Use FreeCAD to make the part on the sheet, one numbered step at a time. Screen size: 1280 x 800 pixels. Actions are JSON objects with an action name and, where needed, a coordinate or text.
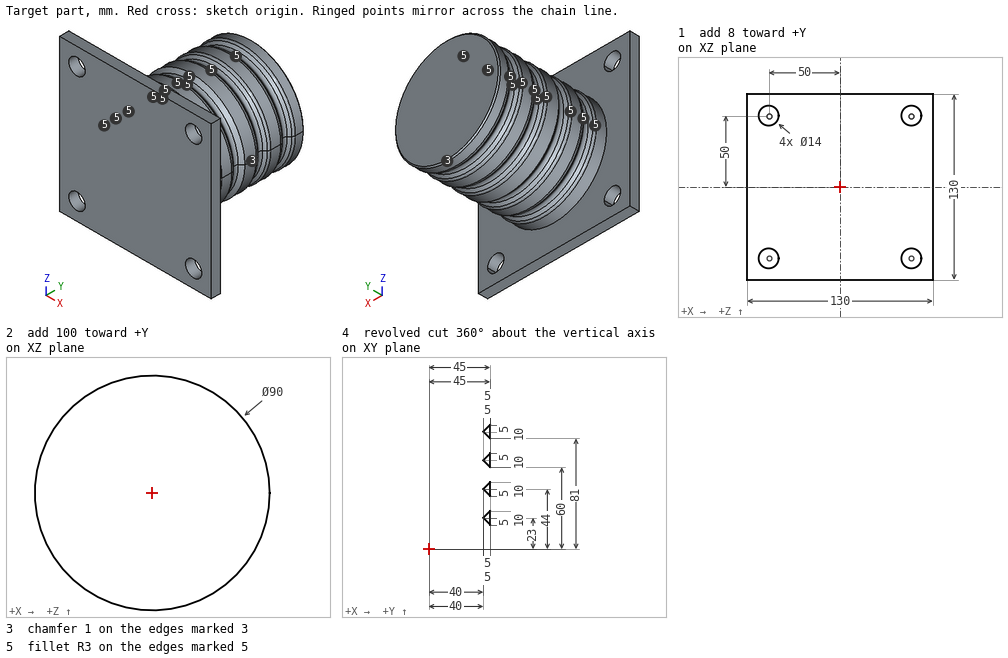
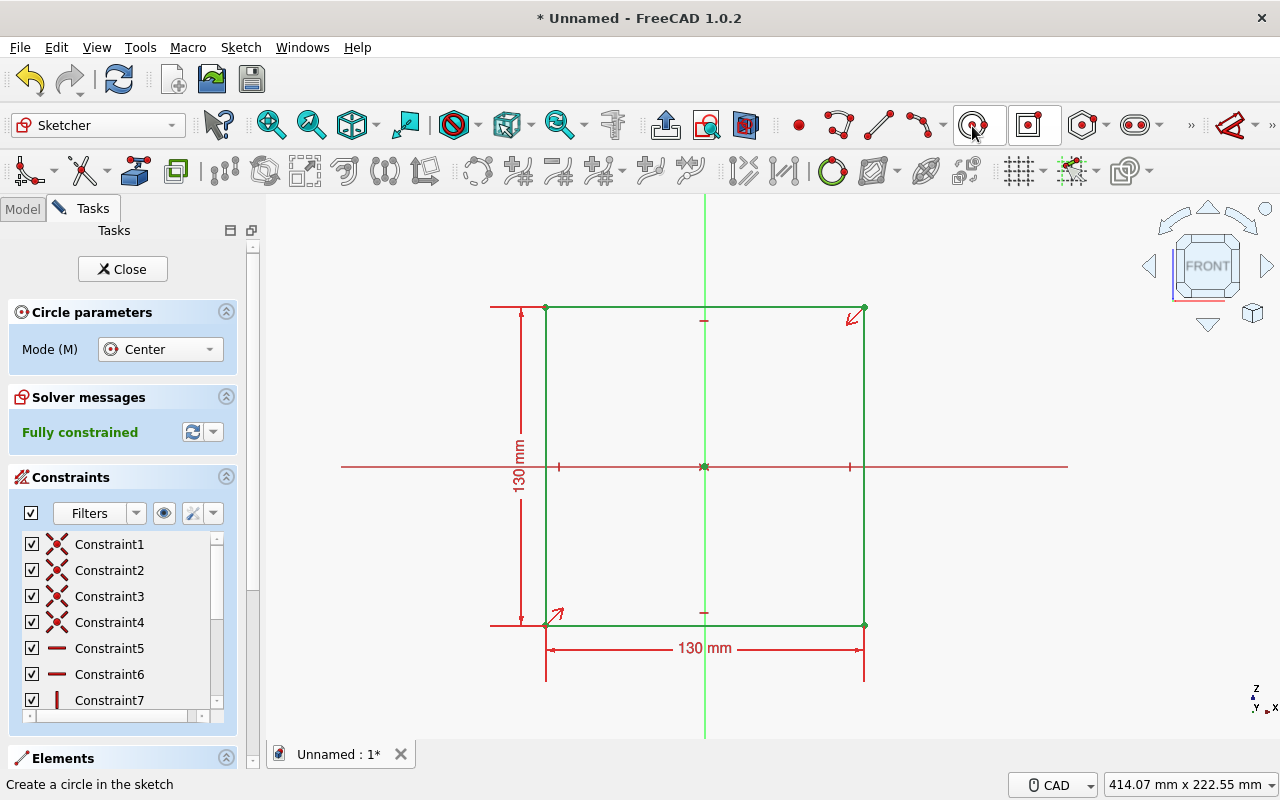
{"action": "scroll", "coordinate": [582, 344], "scroll_direction": "up", "scroll_amount": 2}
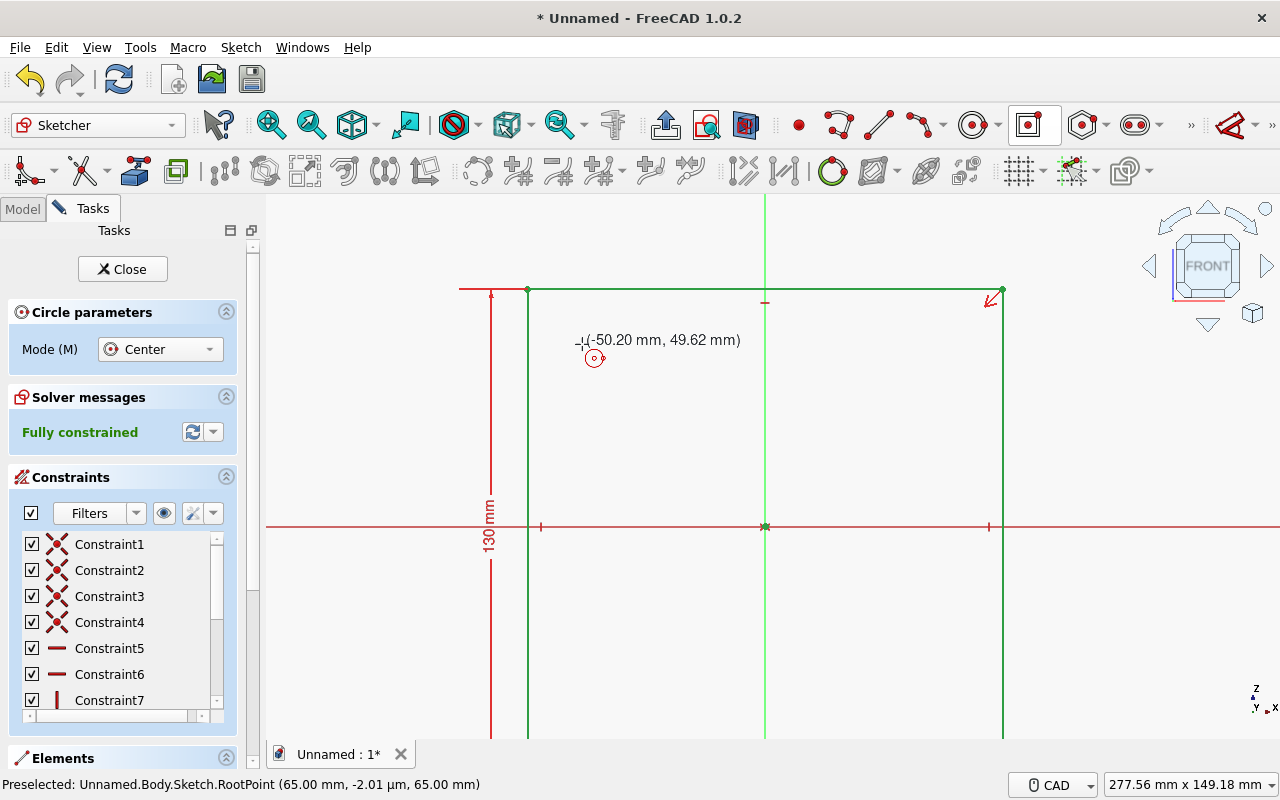
{"action": "left_click", "coordinate": [583, 344]}
{"action": "mouse_move", "coordinate": [601, 326]}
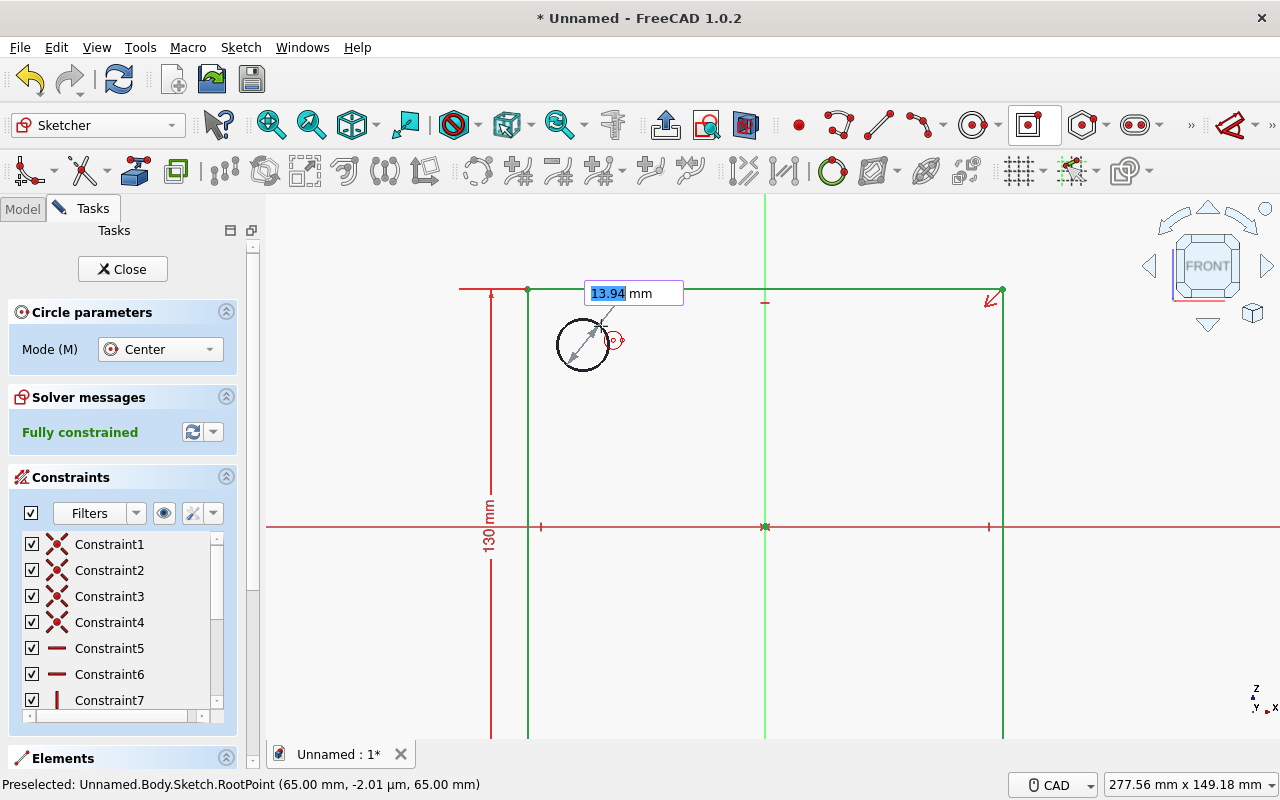
{"action": "type", "text": "14"}
{"action": "key", "text": "Return"}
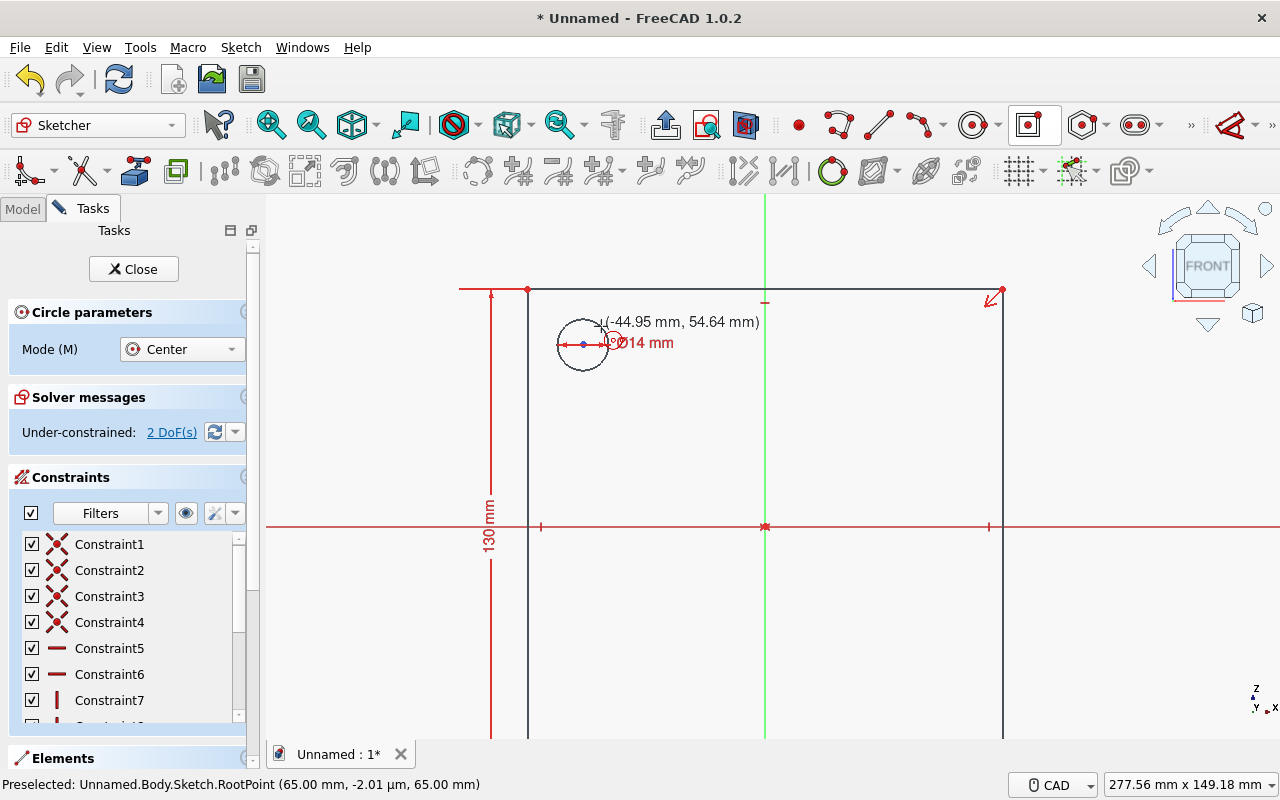
{"action": "left_click", "coordinate": [948, 344]}
{"action": "mouse_move", "coordinate": [966, 326]}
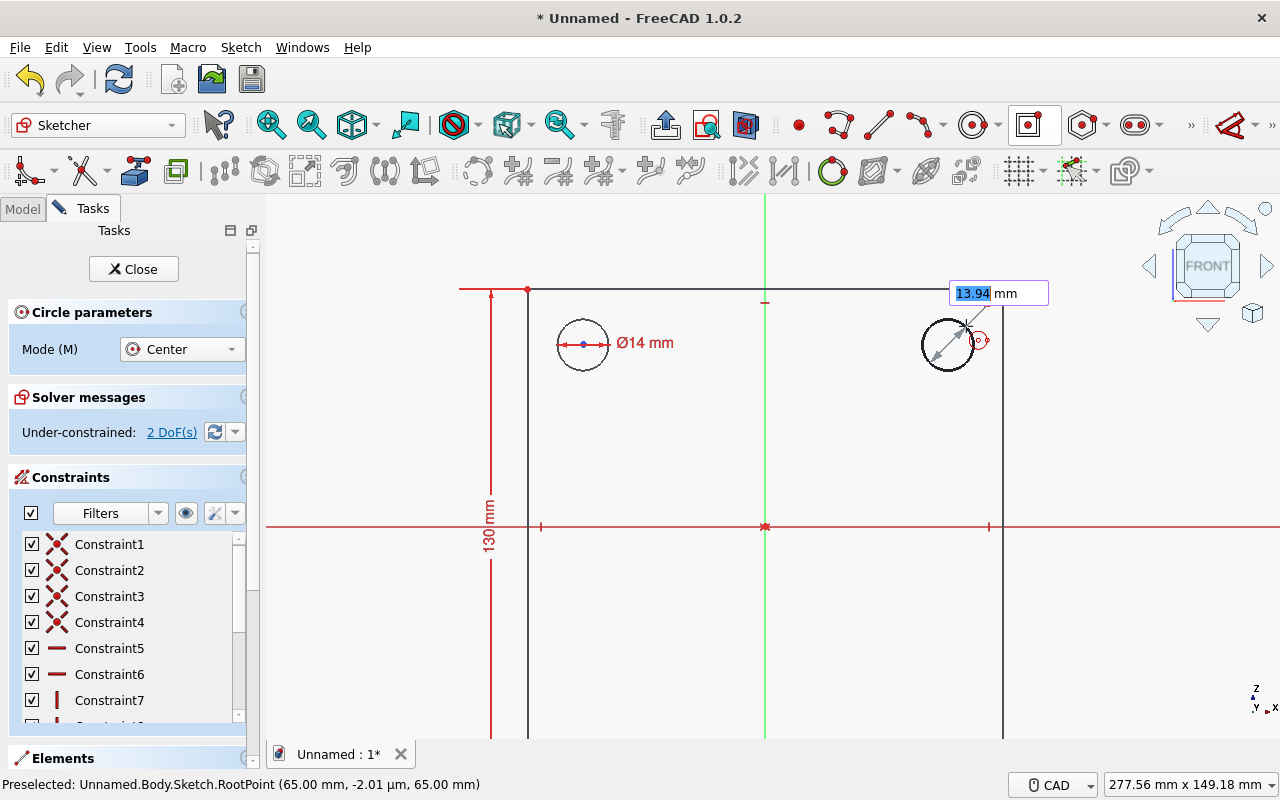
{"action": "type", "text": "14"}
{"action": "key", "text": "Return"}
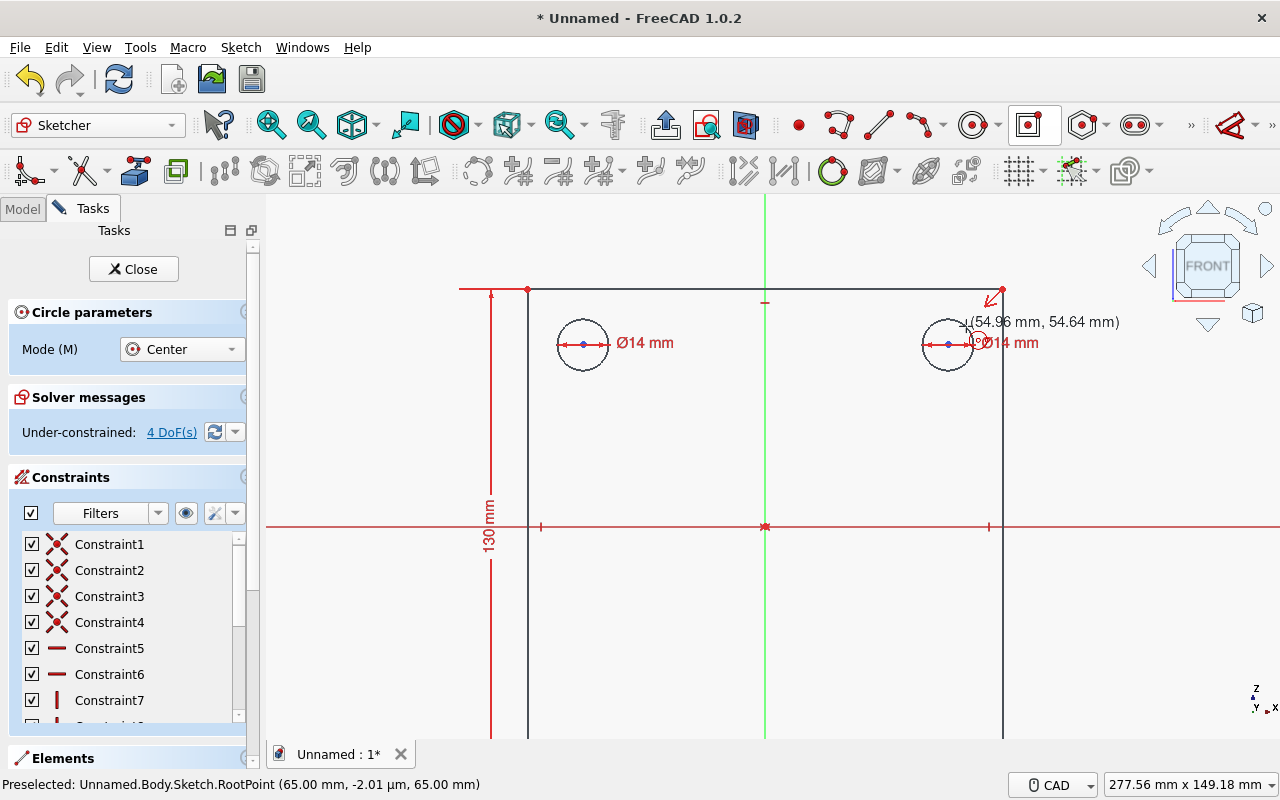
{"action": "left_click", "coordinate": [583, 709]}
{"action": "mouse_move", "coordinate": [601, 691]}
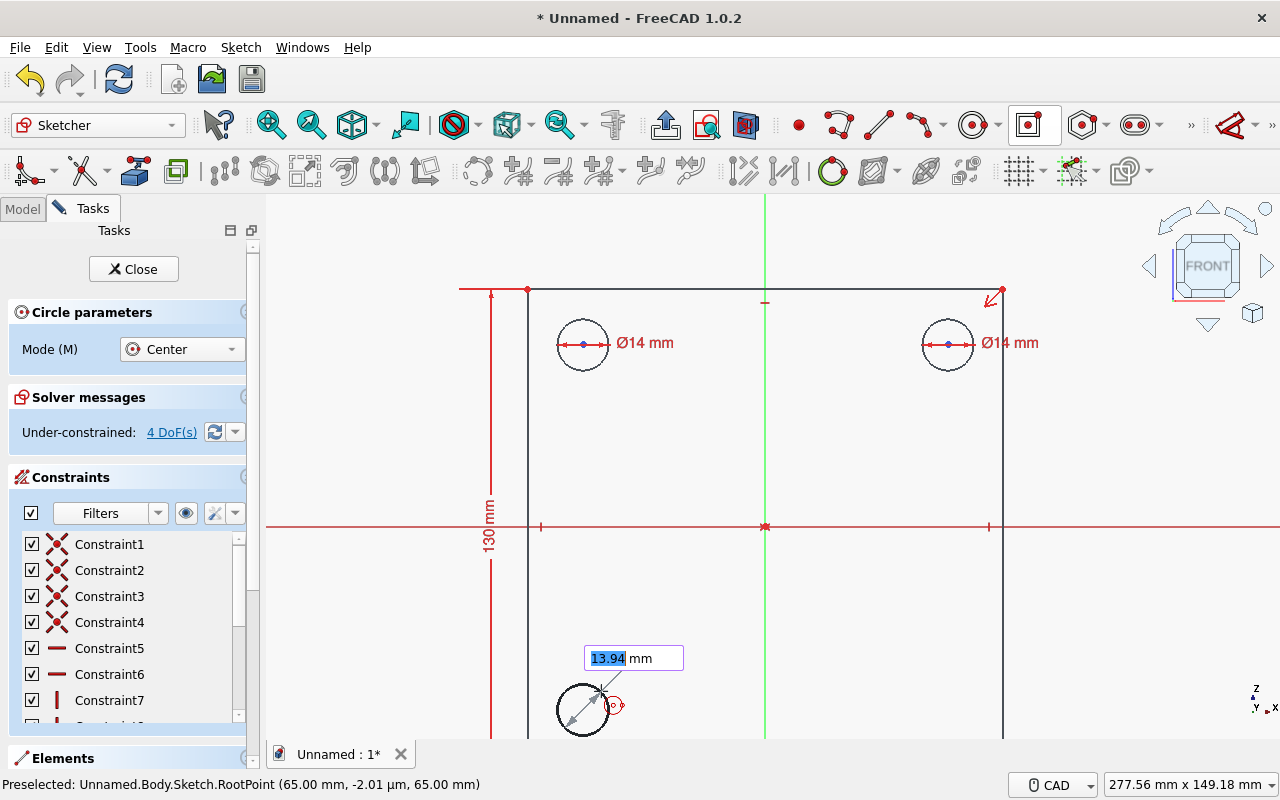
{"action": "type", "text": "14"}
{"action": "key", "text": "Return"}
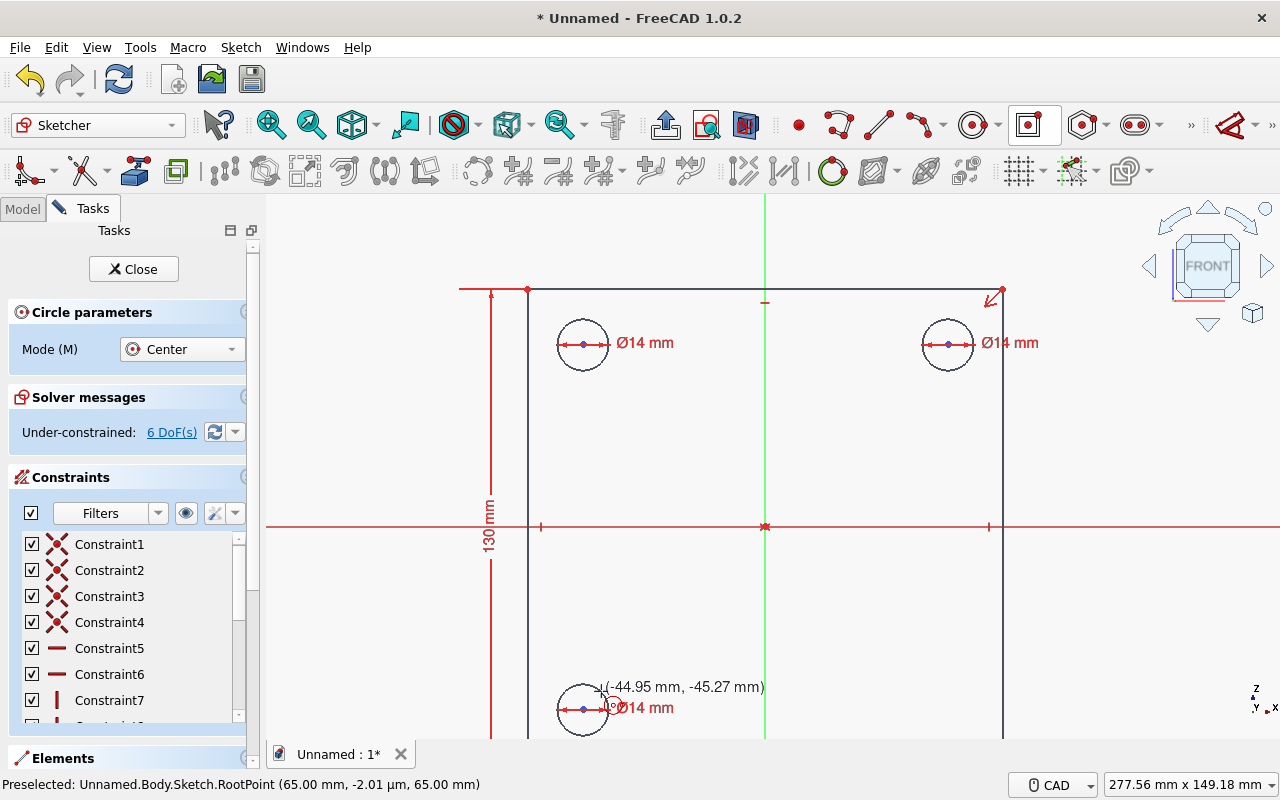
{"action": "left_click", "coordinate": [948, 709]}
{"action": "mouse_move", "coordinate": [966, 691]}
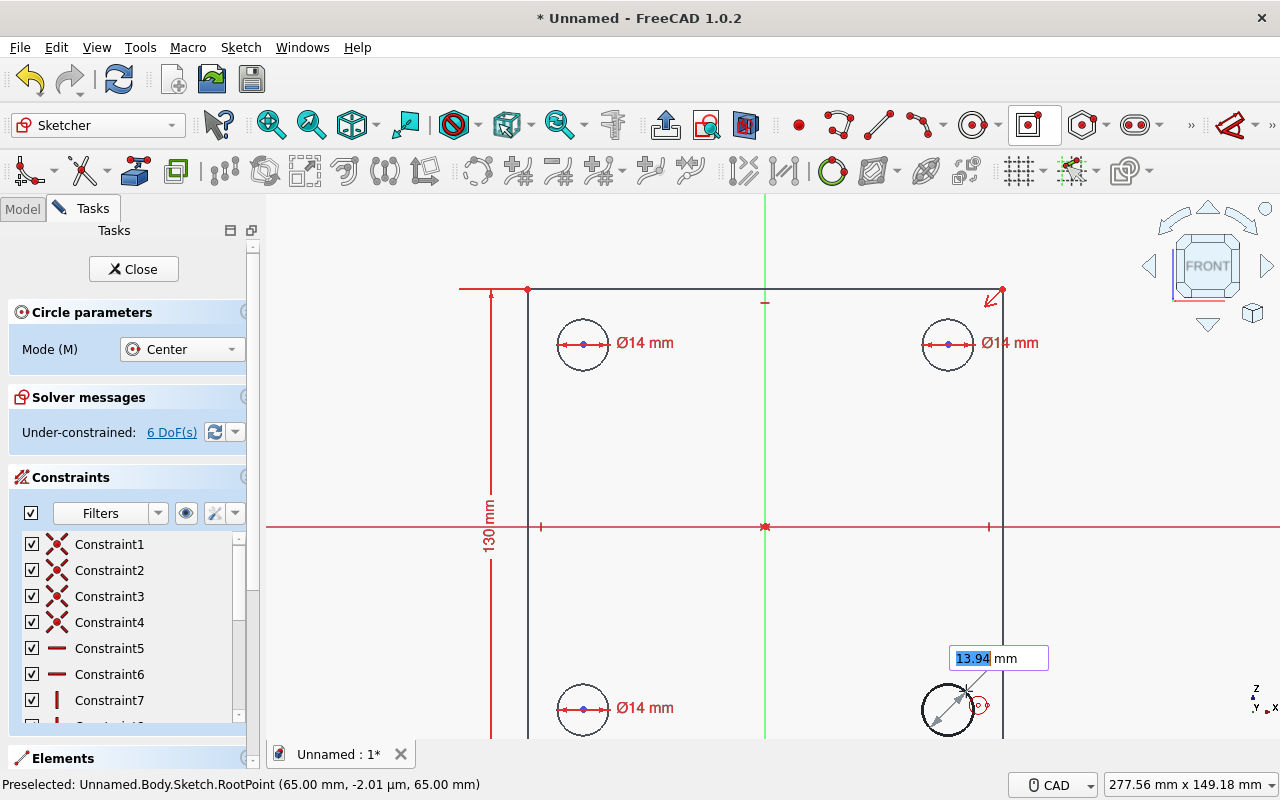
{"action": "type", "text": "14"}
{"action": "key", "text": "Return"}
{"action": "key", "text": "Escape"}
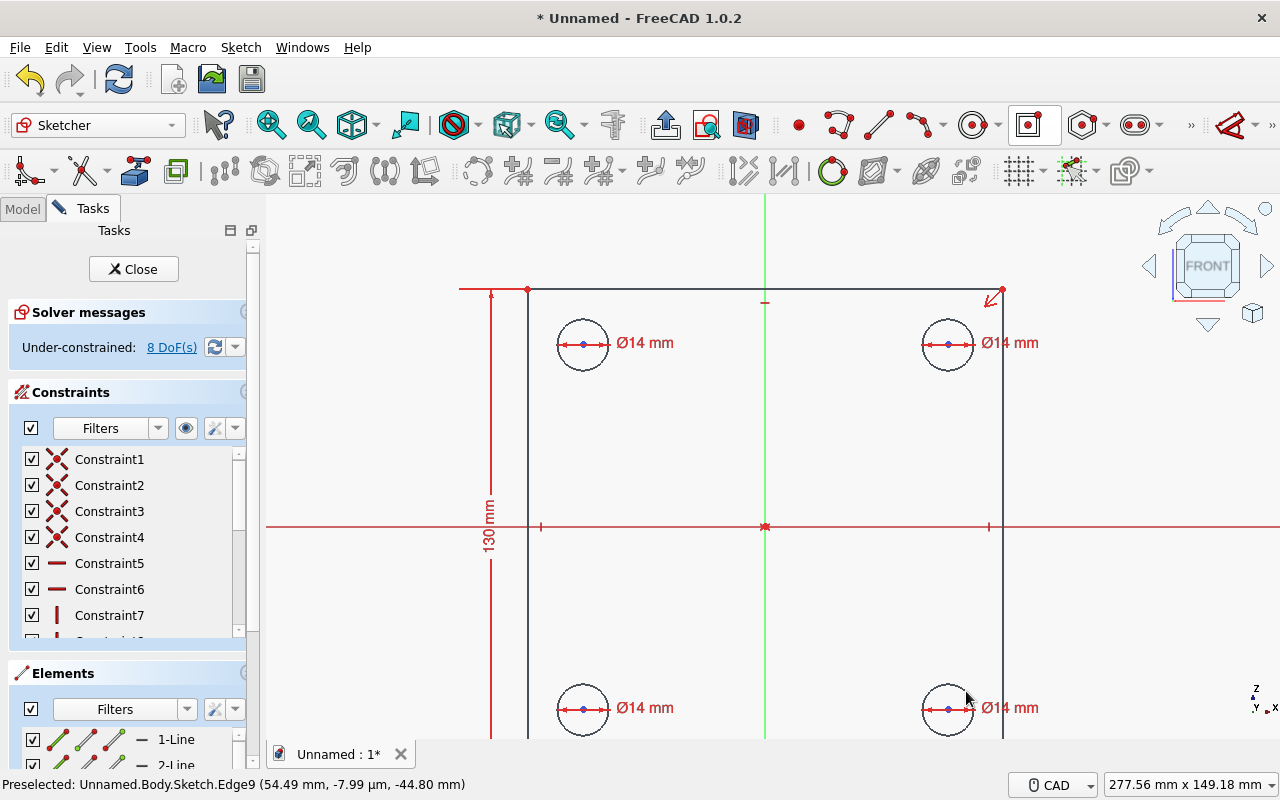
{"action": "left_click", "coordinate": [583, 345]}